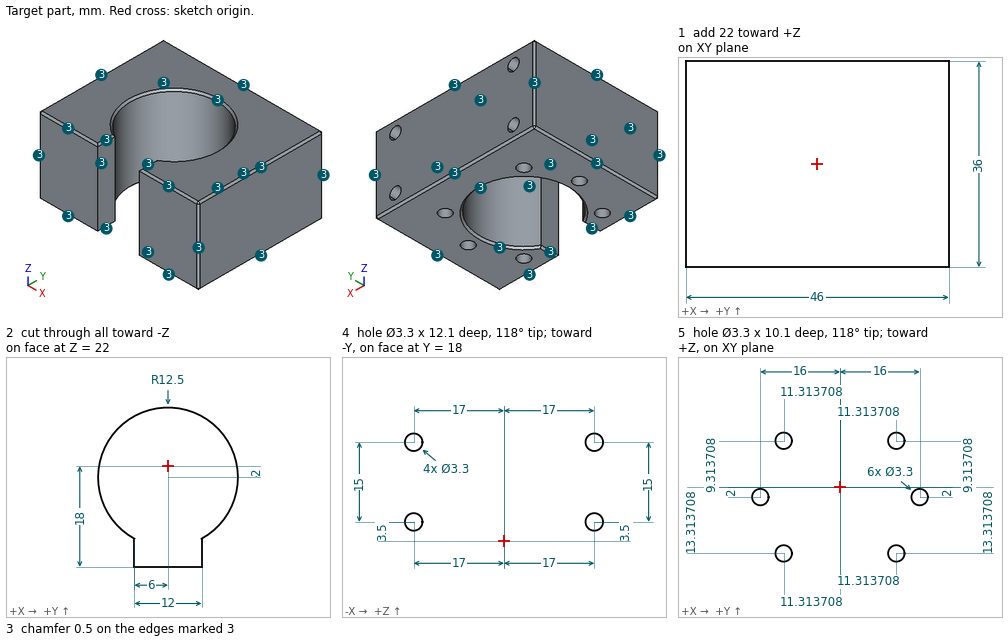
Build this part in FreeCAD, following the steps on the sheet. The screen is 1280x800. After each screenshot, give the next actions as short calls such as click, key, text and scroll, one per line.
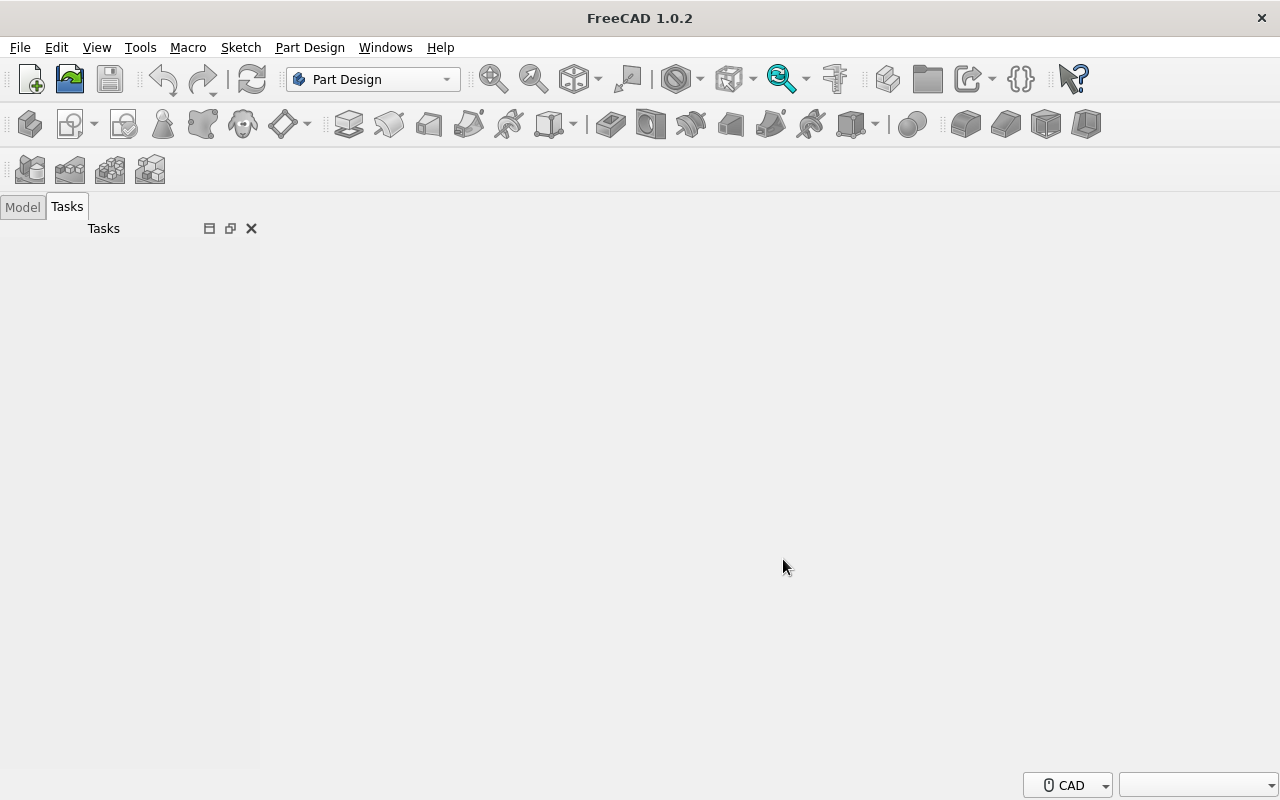
click(30, 80)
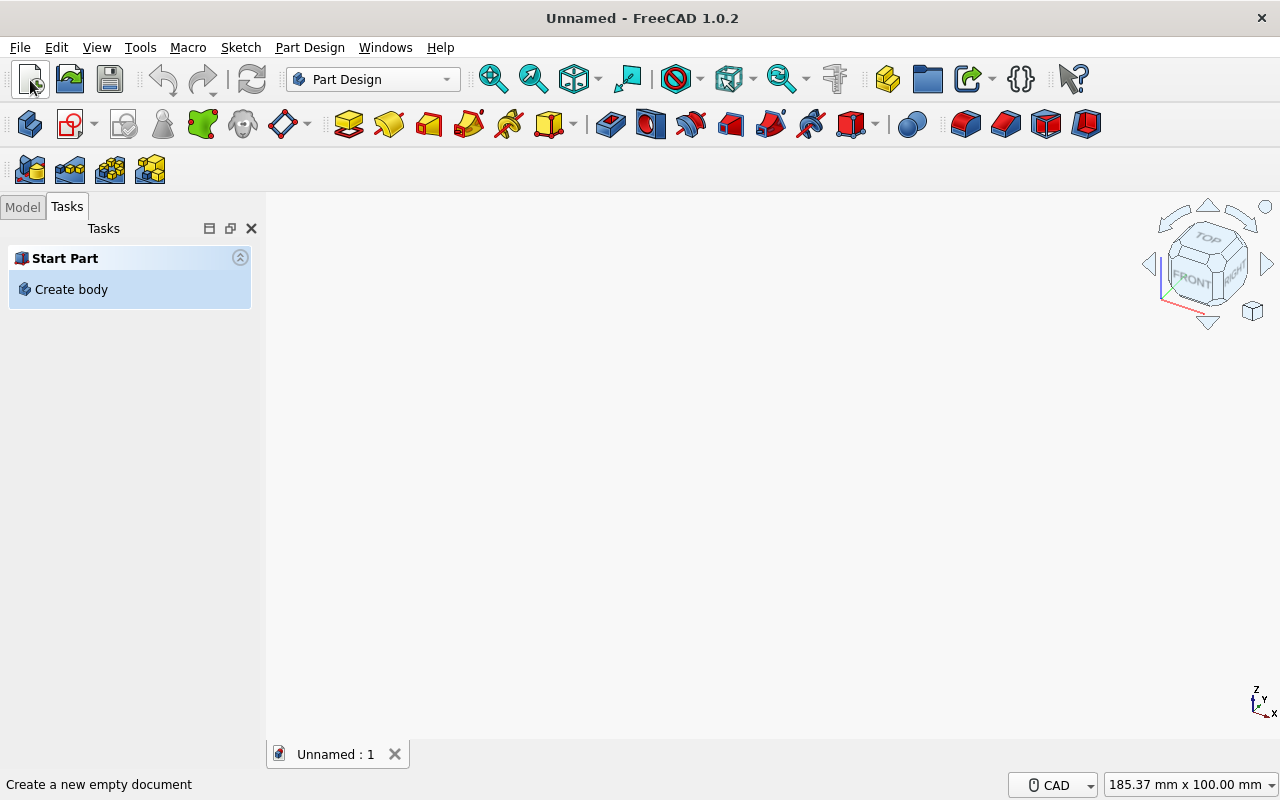
click(70, 124)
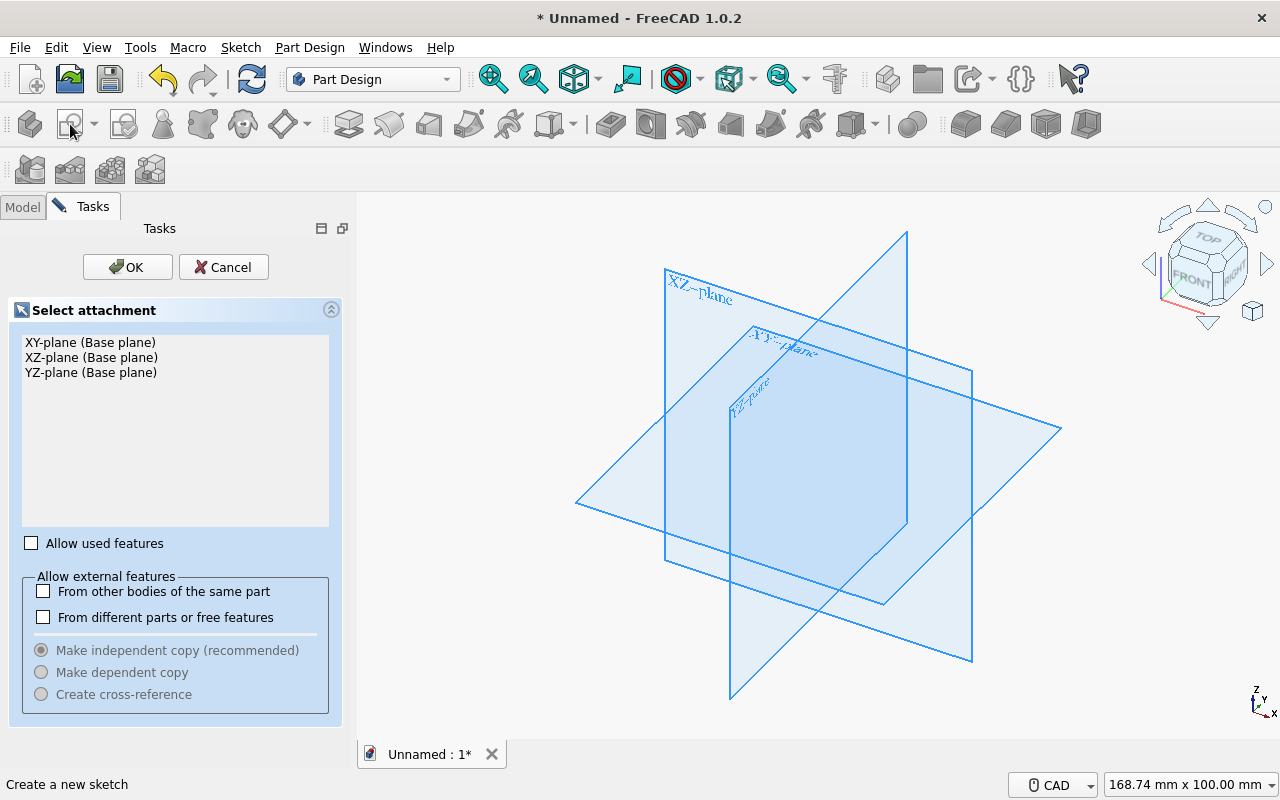
click(82, 342)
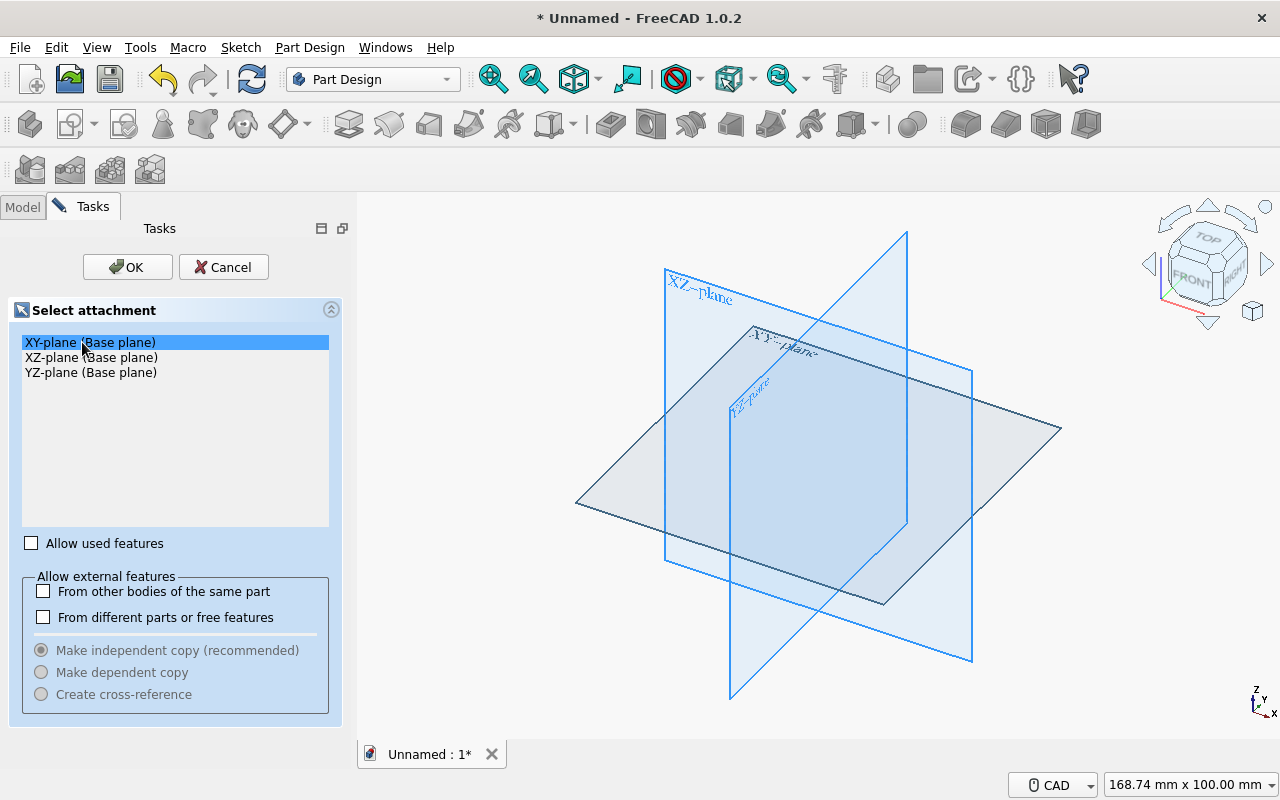
click(128, 267)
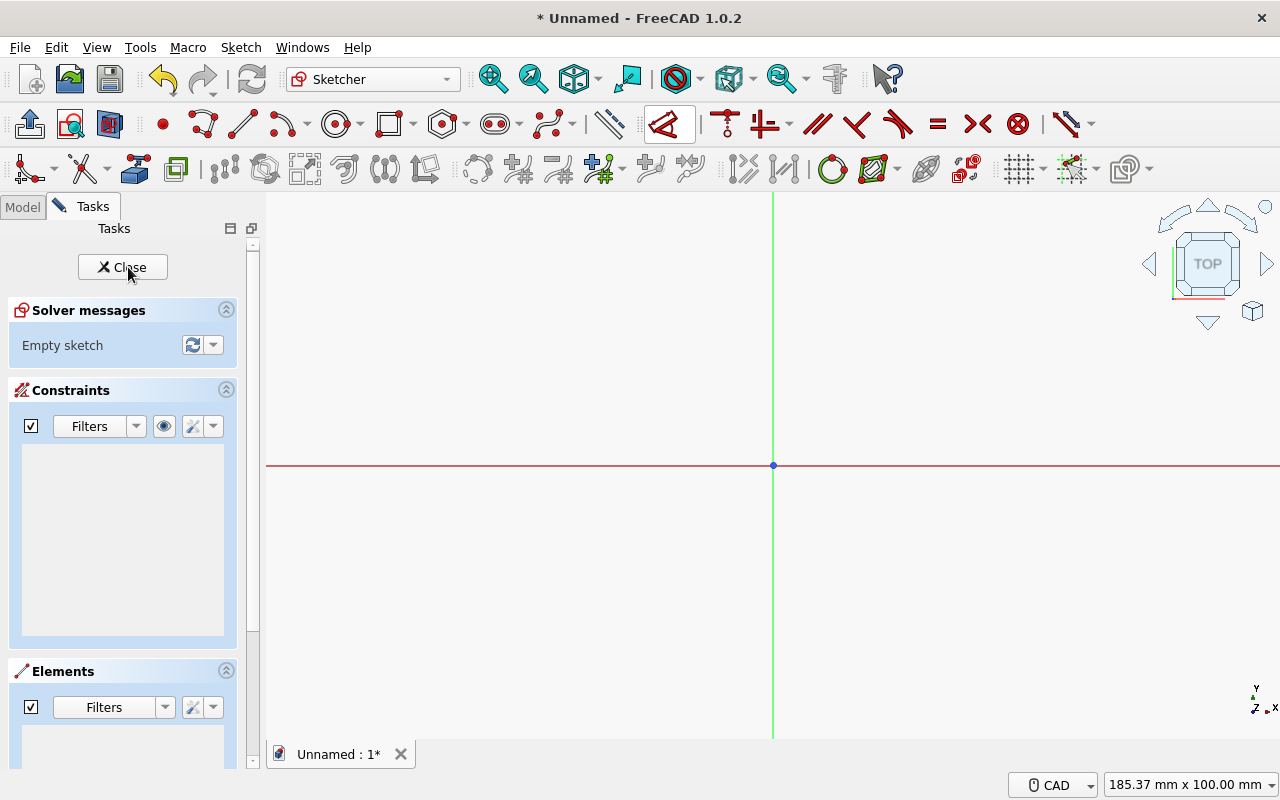
scroll(856, 466, up, 3)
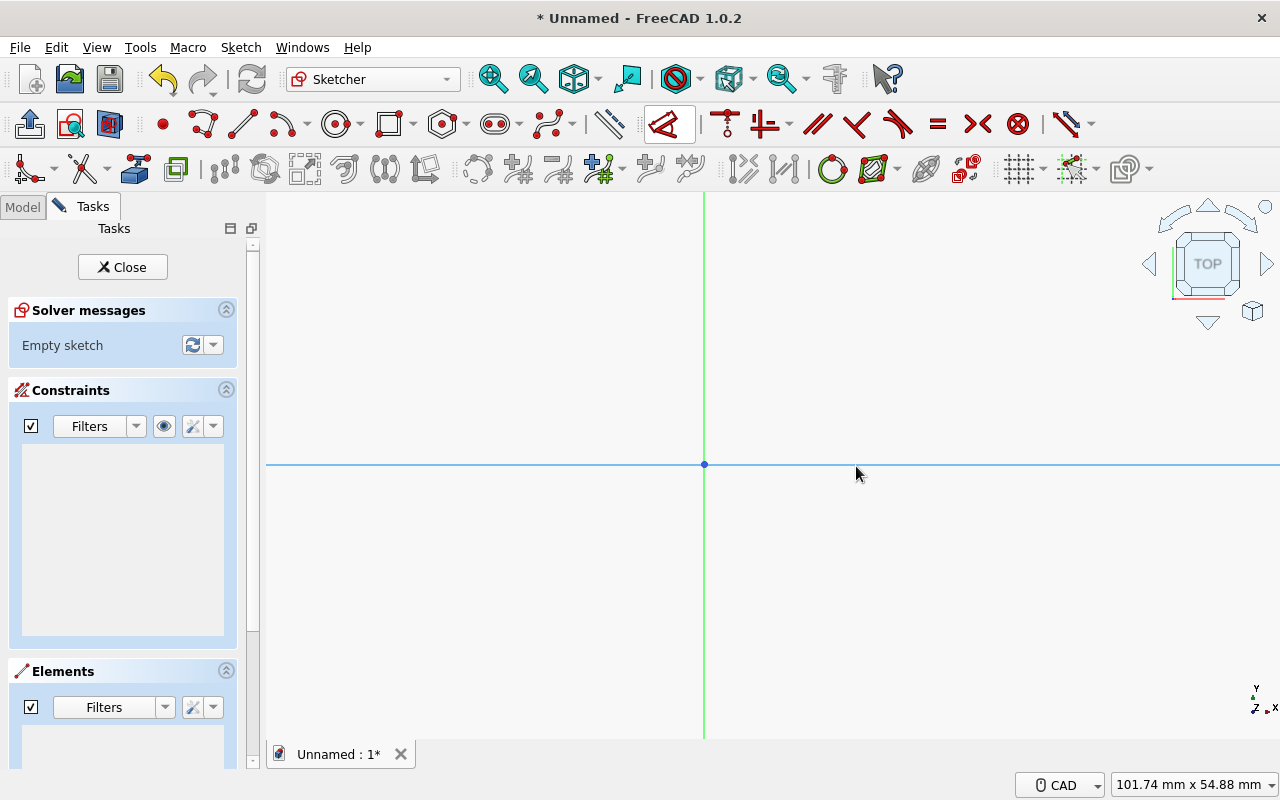
key(g)
key(v)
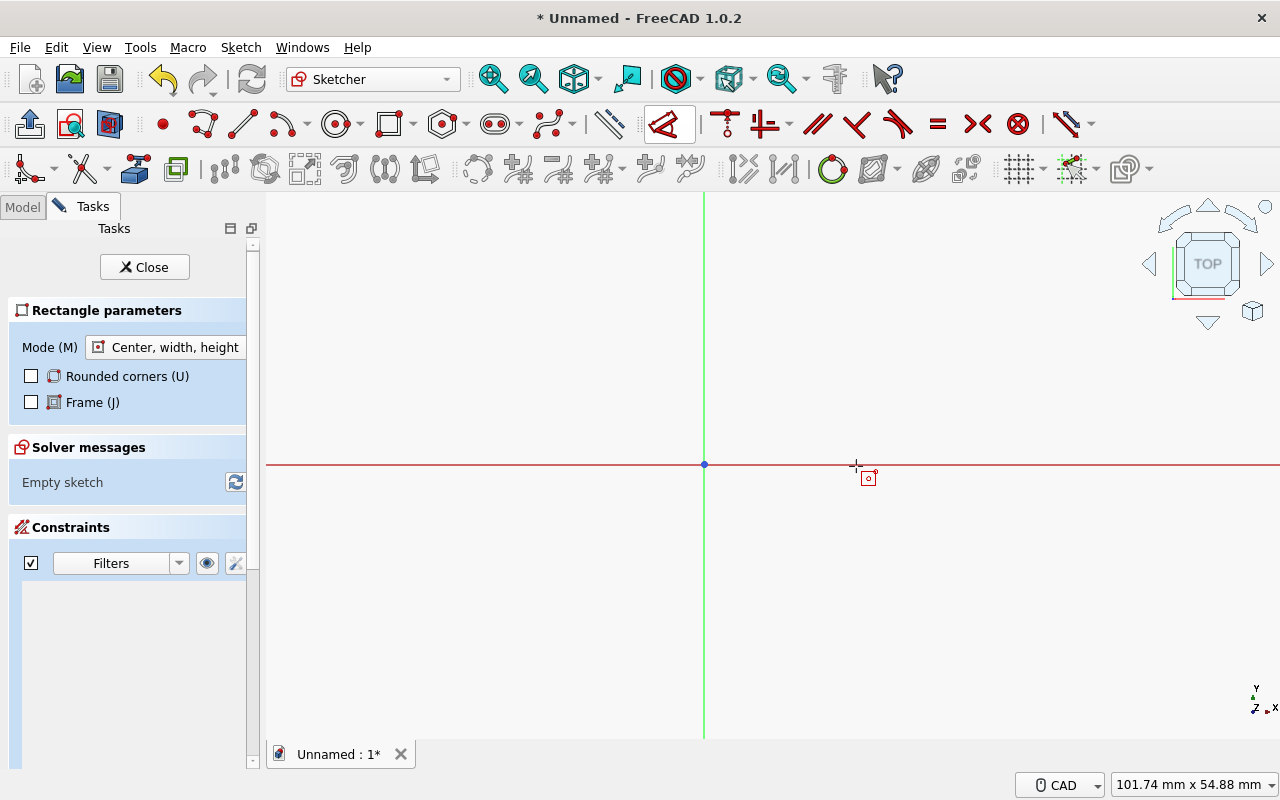
click(704, 465)
move(934, 285)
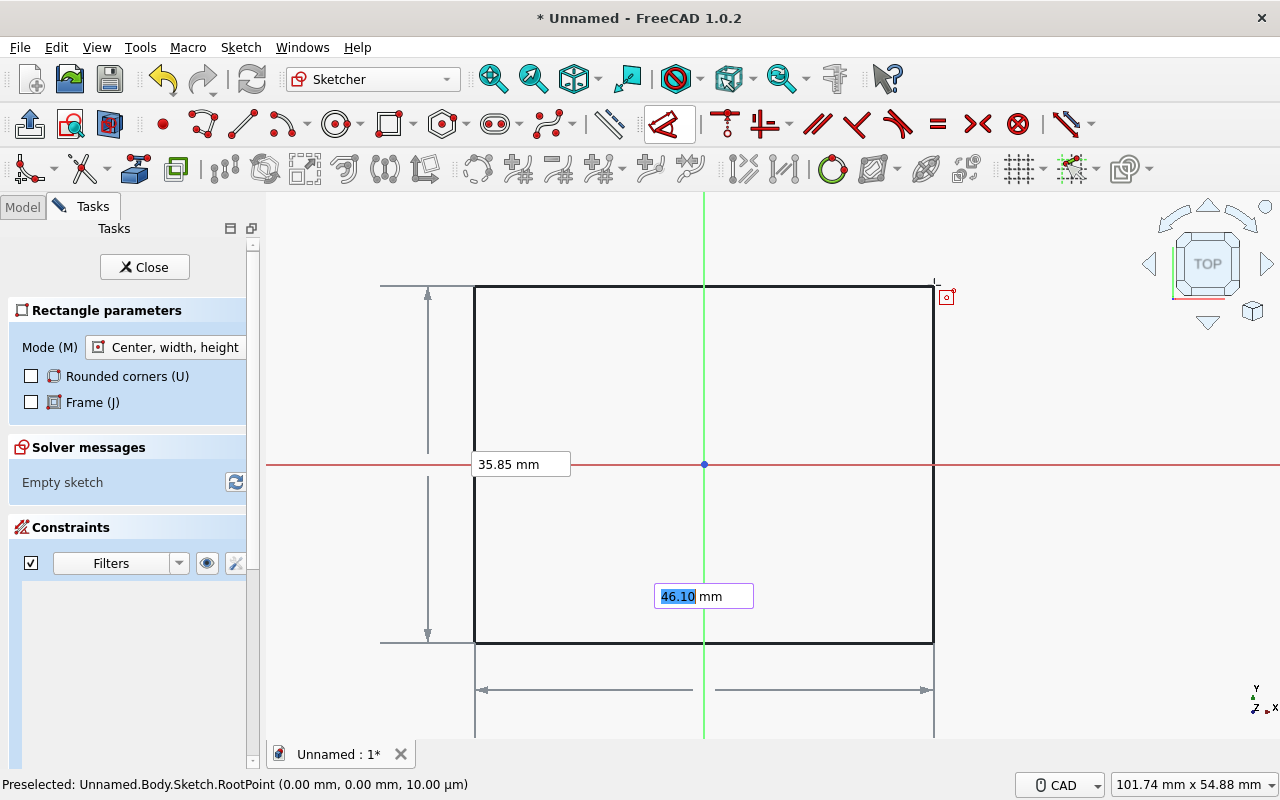
text(46)
key(Tab)
text(36)
key(Return)
key(Escape)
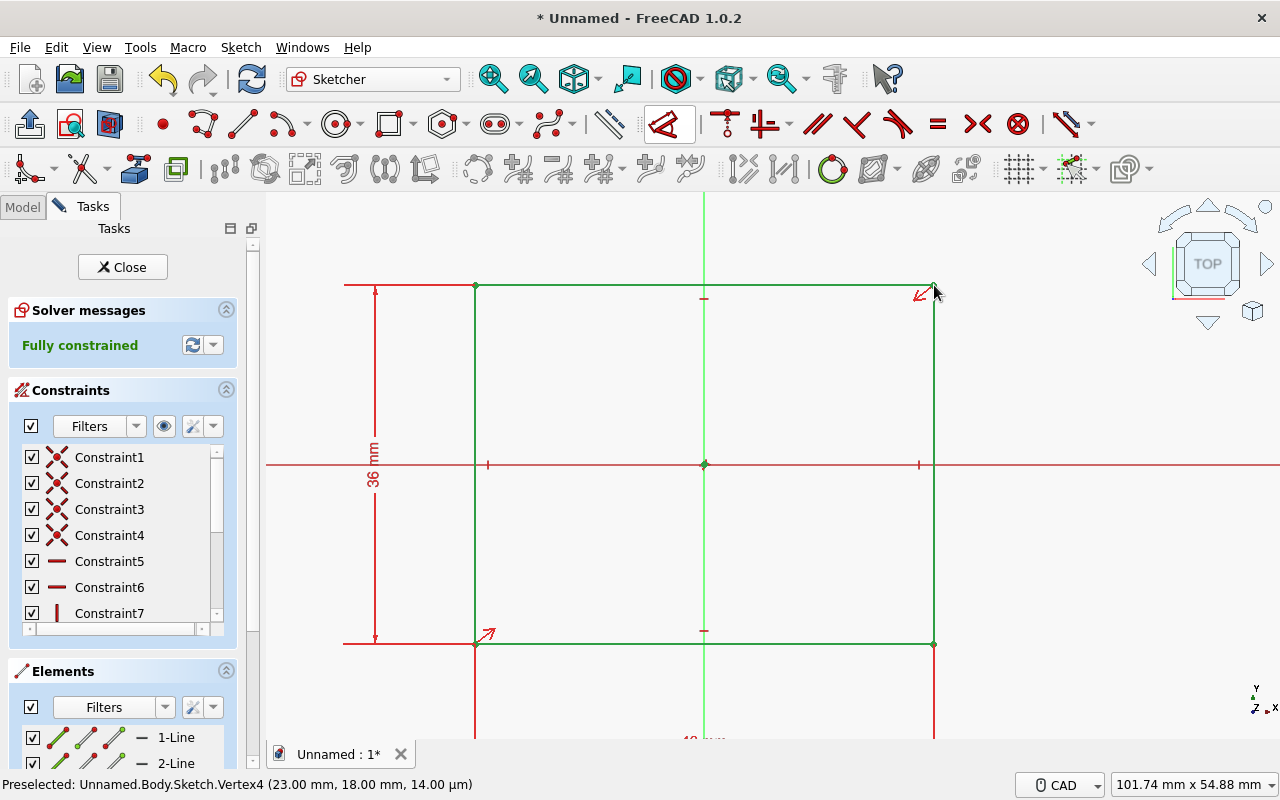
click(123, 267)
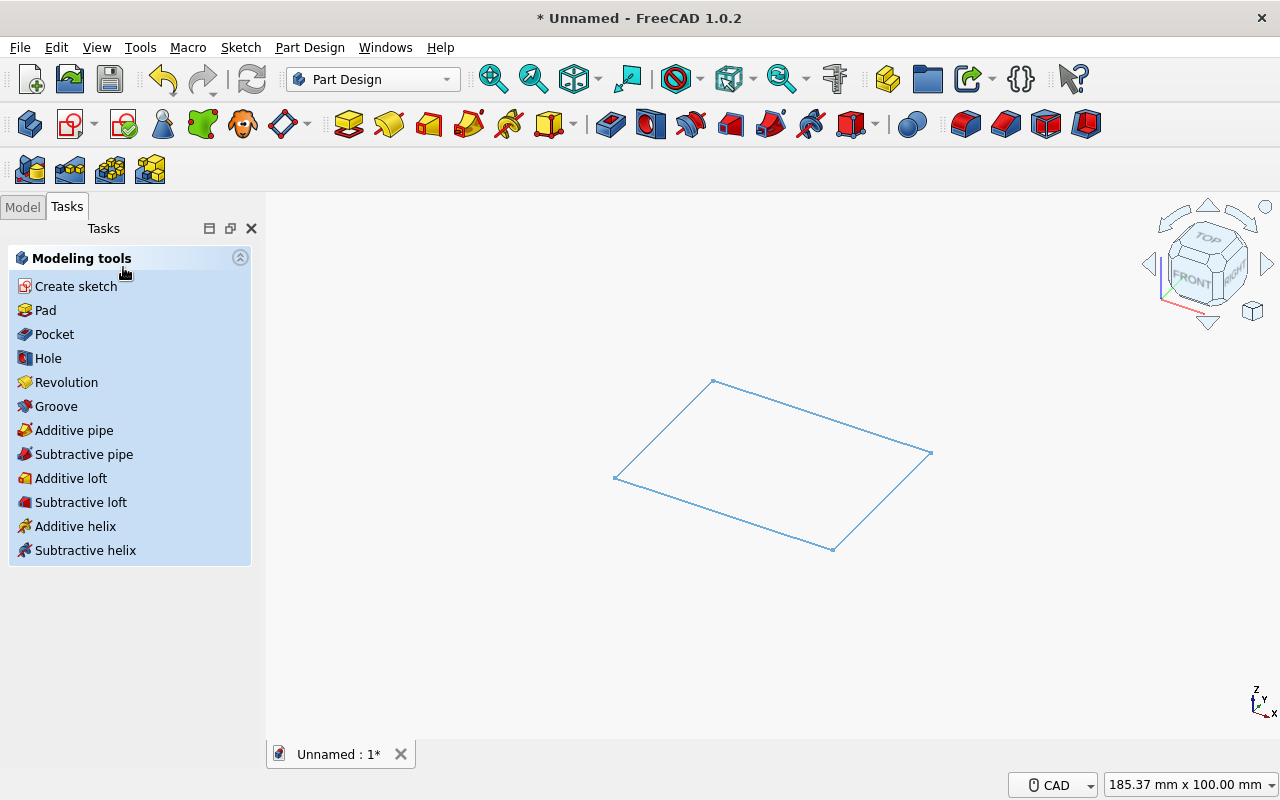
click(350, 124)